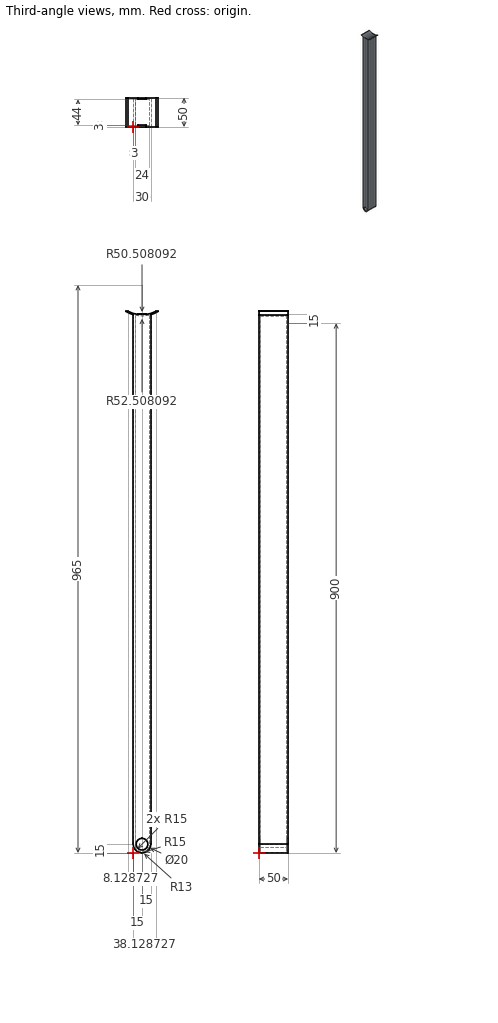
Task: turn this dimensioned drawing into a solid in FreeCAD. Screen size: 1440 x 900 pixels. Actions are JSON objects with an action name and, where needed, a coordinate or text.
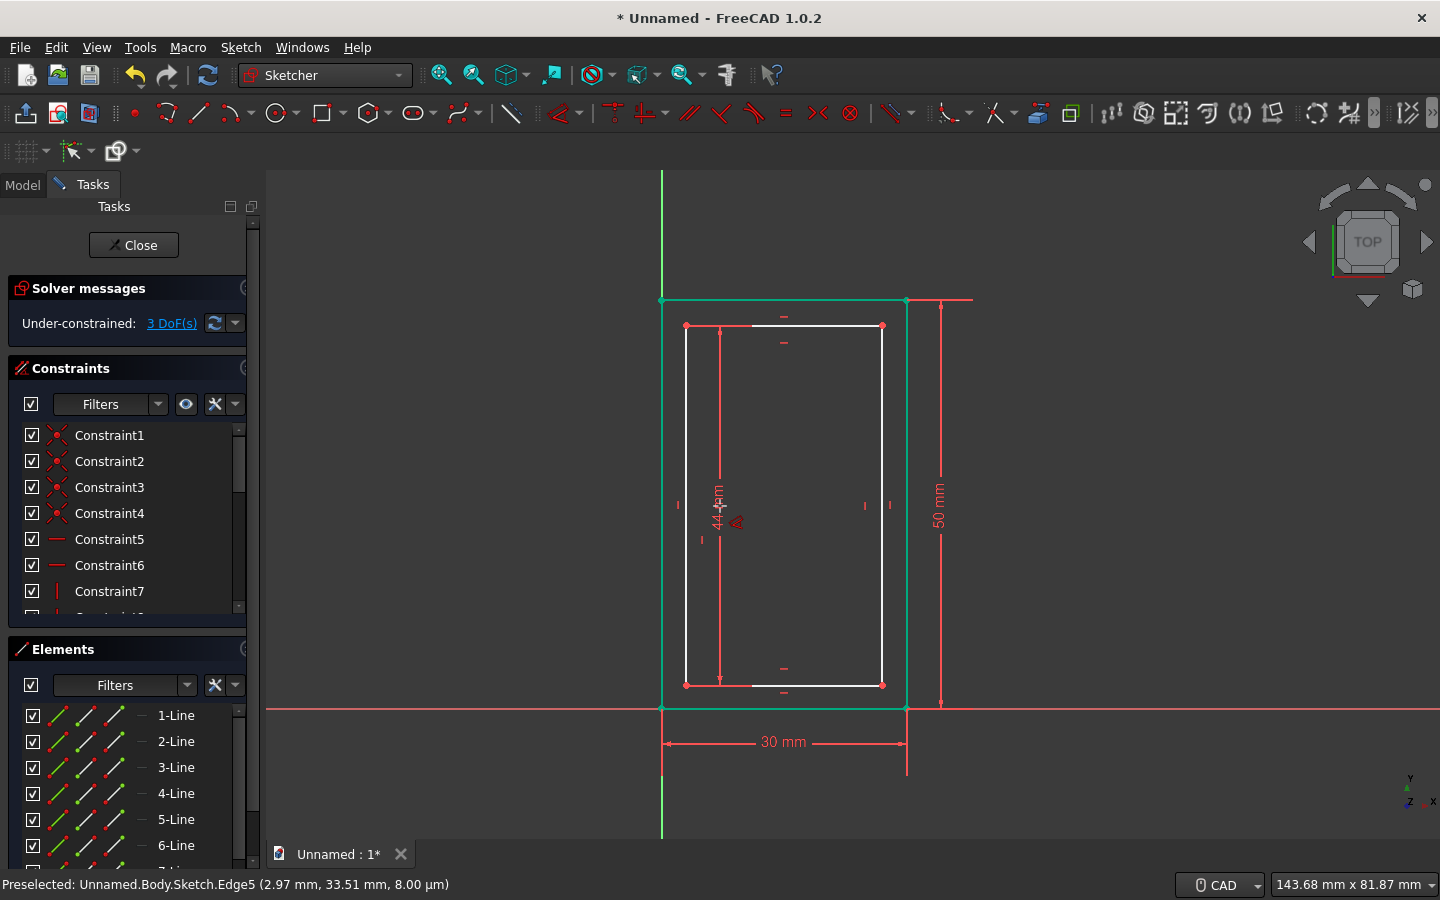
{"action": "left_click", "coordinate": [745, 686]}
{"action": "left_click", "coordinate": [784, 652]}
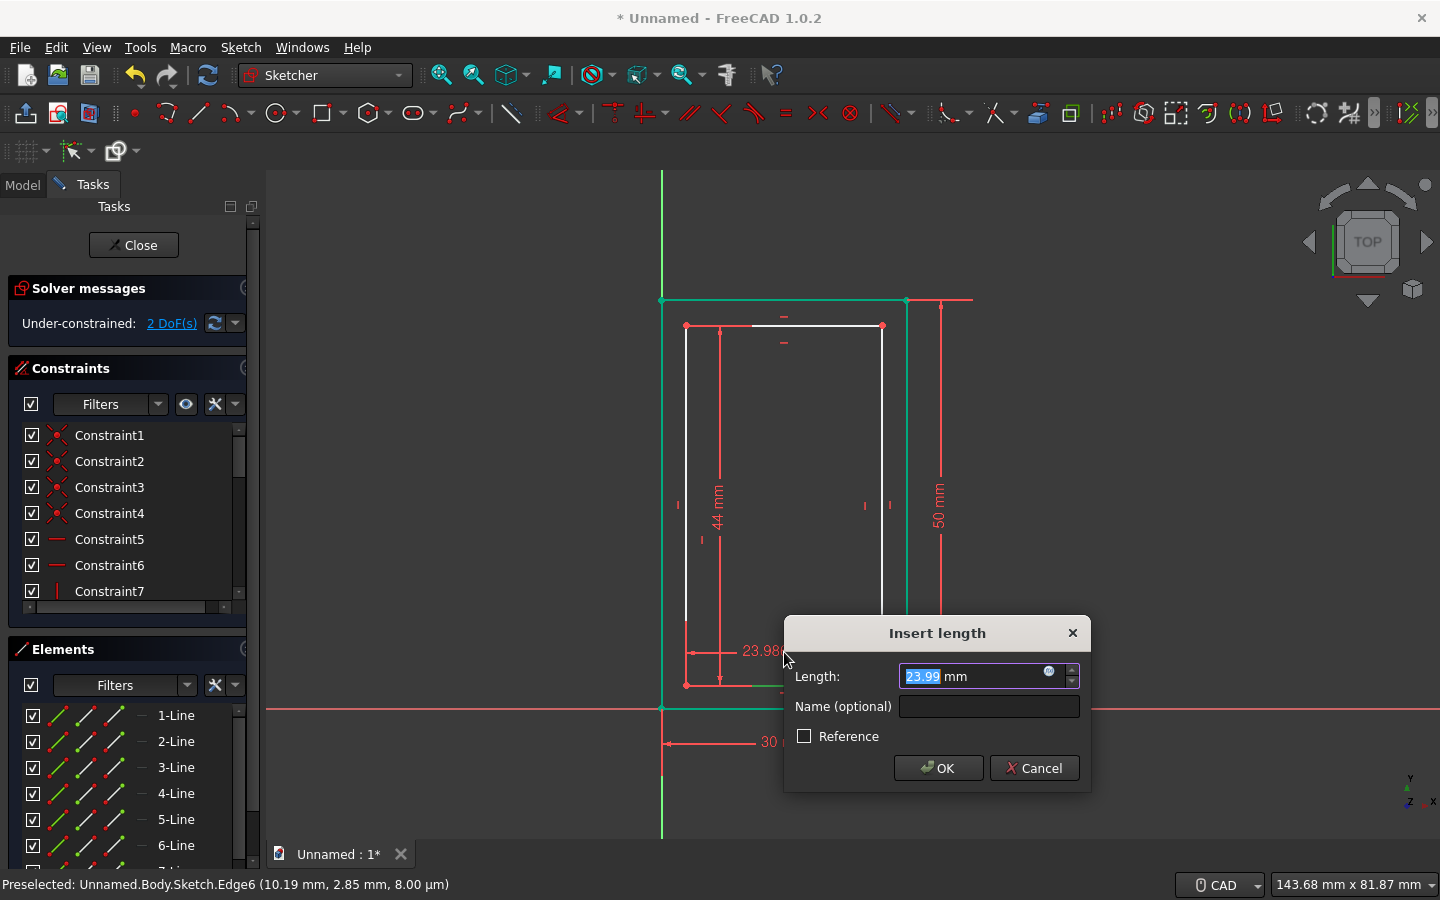
{"action": "type", "text": "24"}
{"action": "key", "text": "Return"}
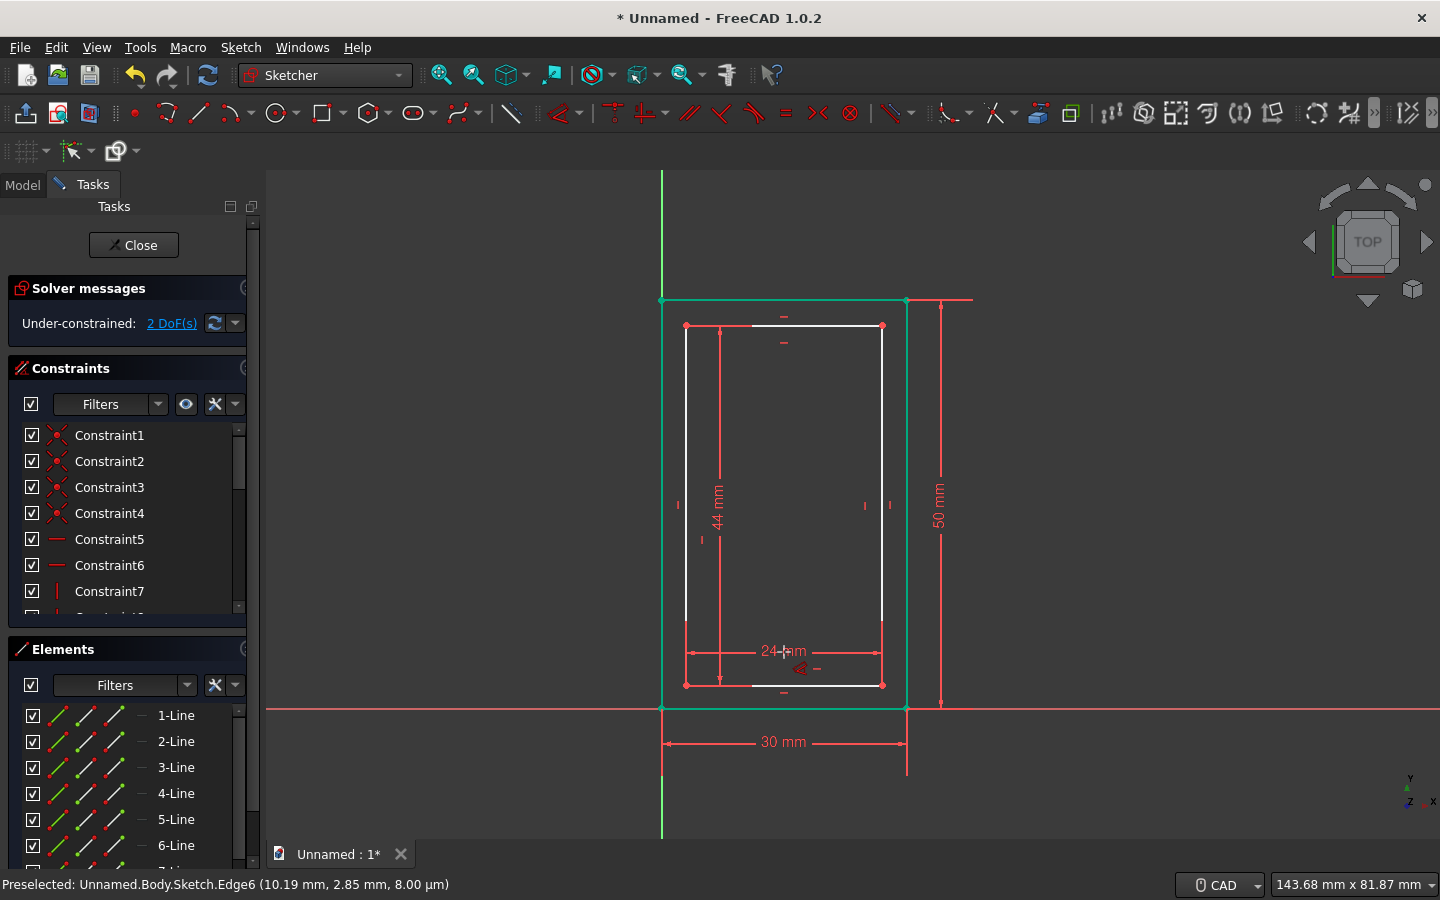
{"action": "scroll", "coordinate": [686, 326], "scroll_direction": "up", "scroll_amount": 3}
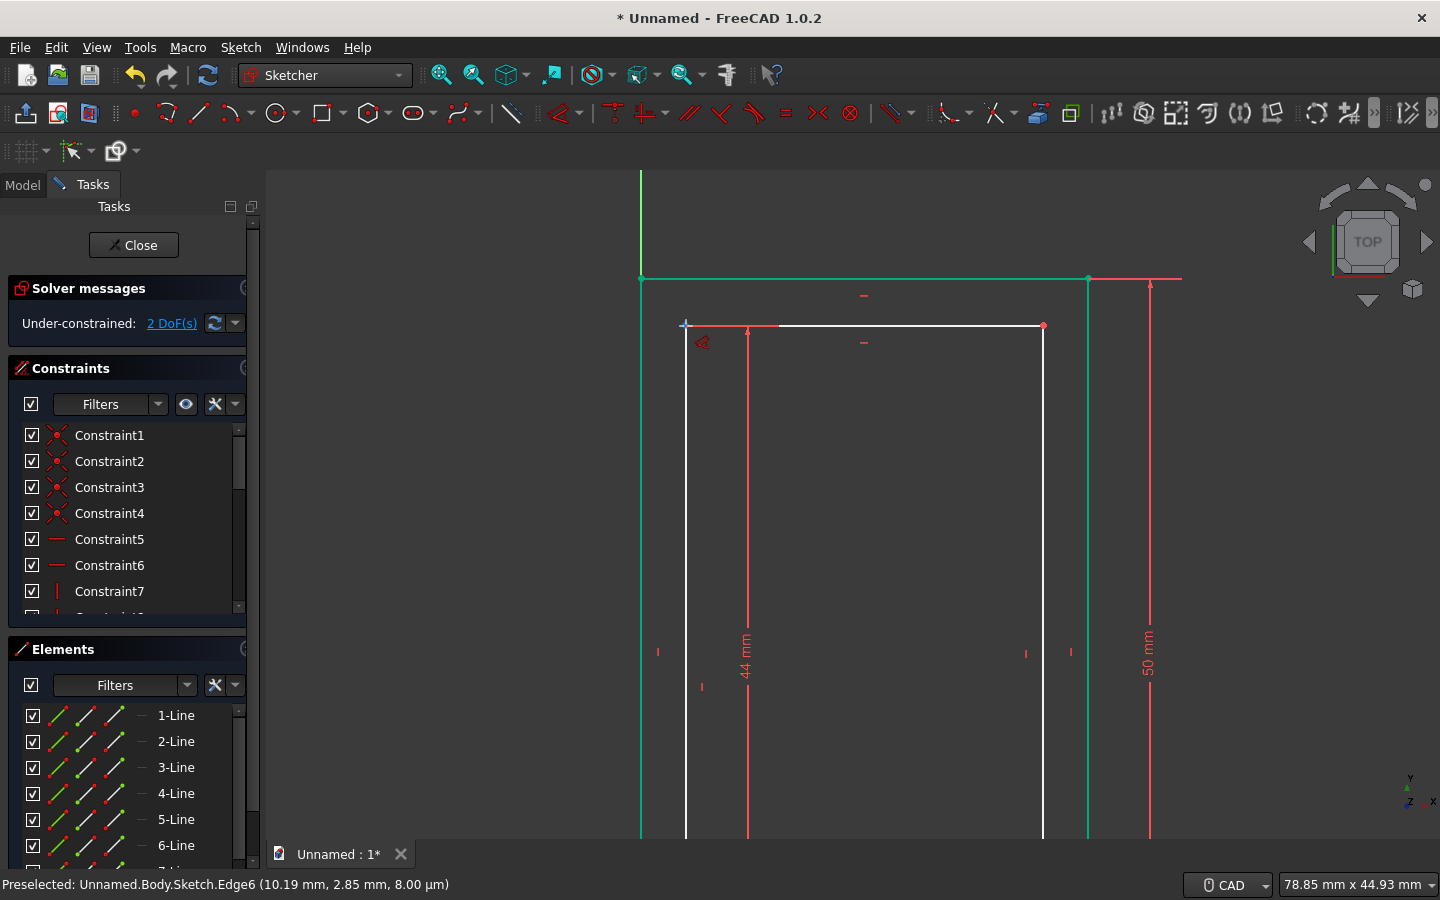
{"action": "left_click", "coordinate": [686, 326]}
{"action": "left_click", "coordinate": [664, 244]}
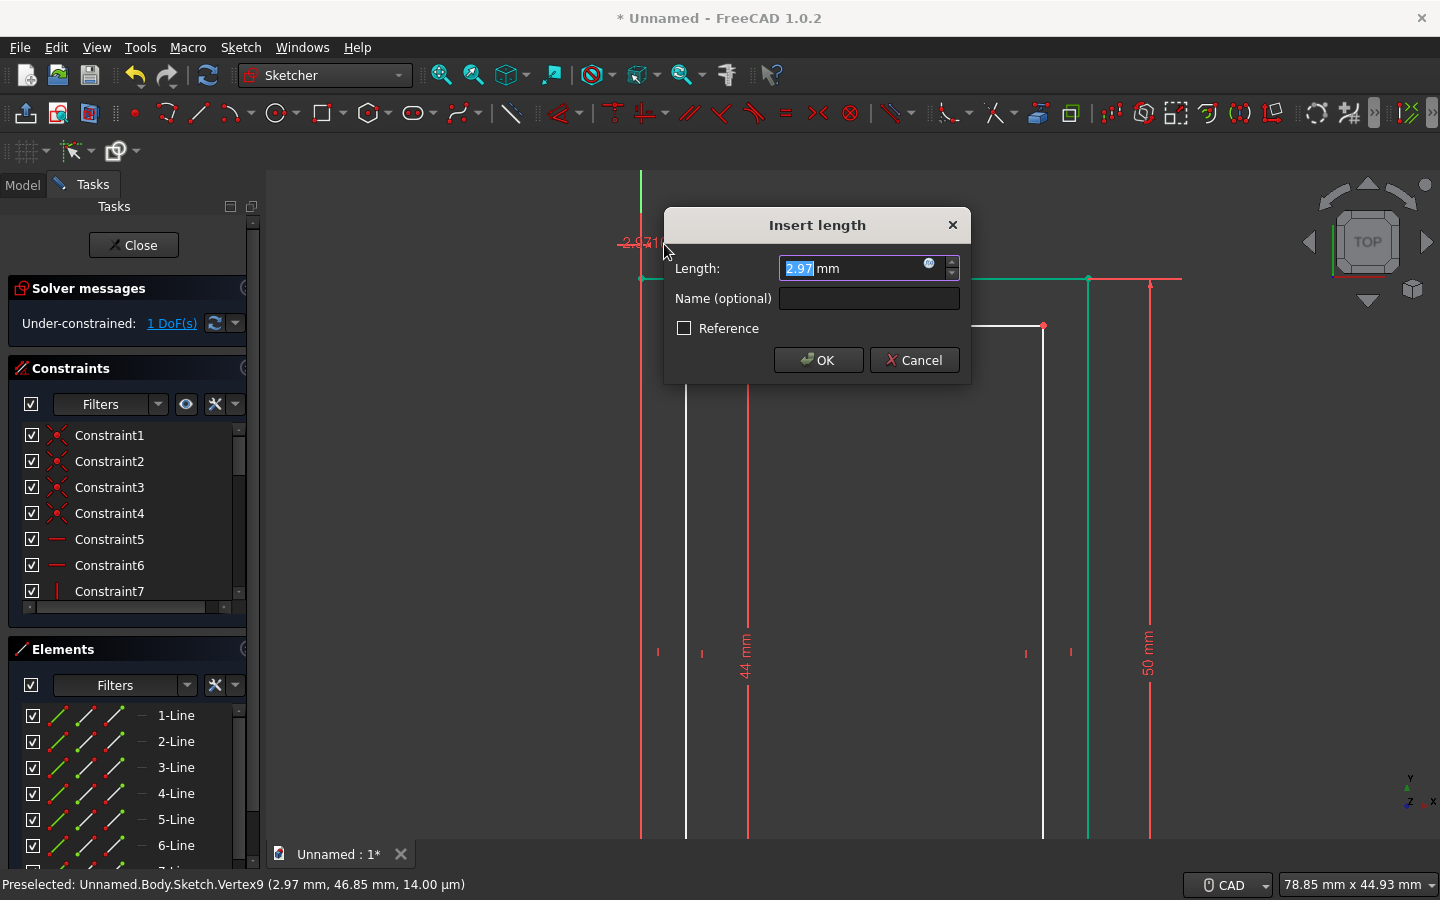
{"action": "type", "text": "3"}
{"action": "key", "text": "Return"}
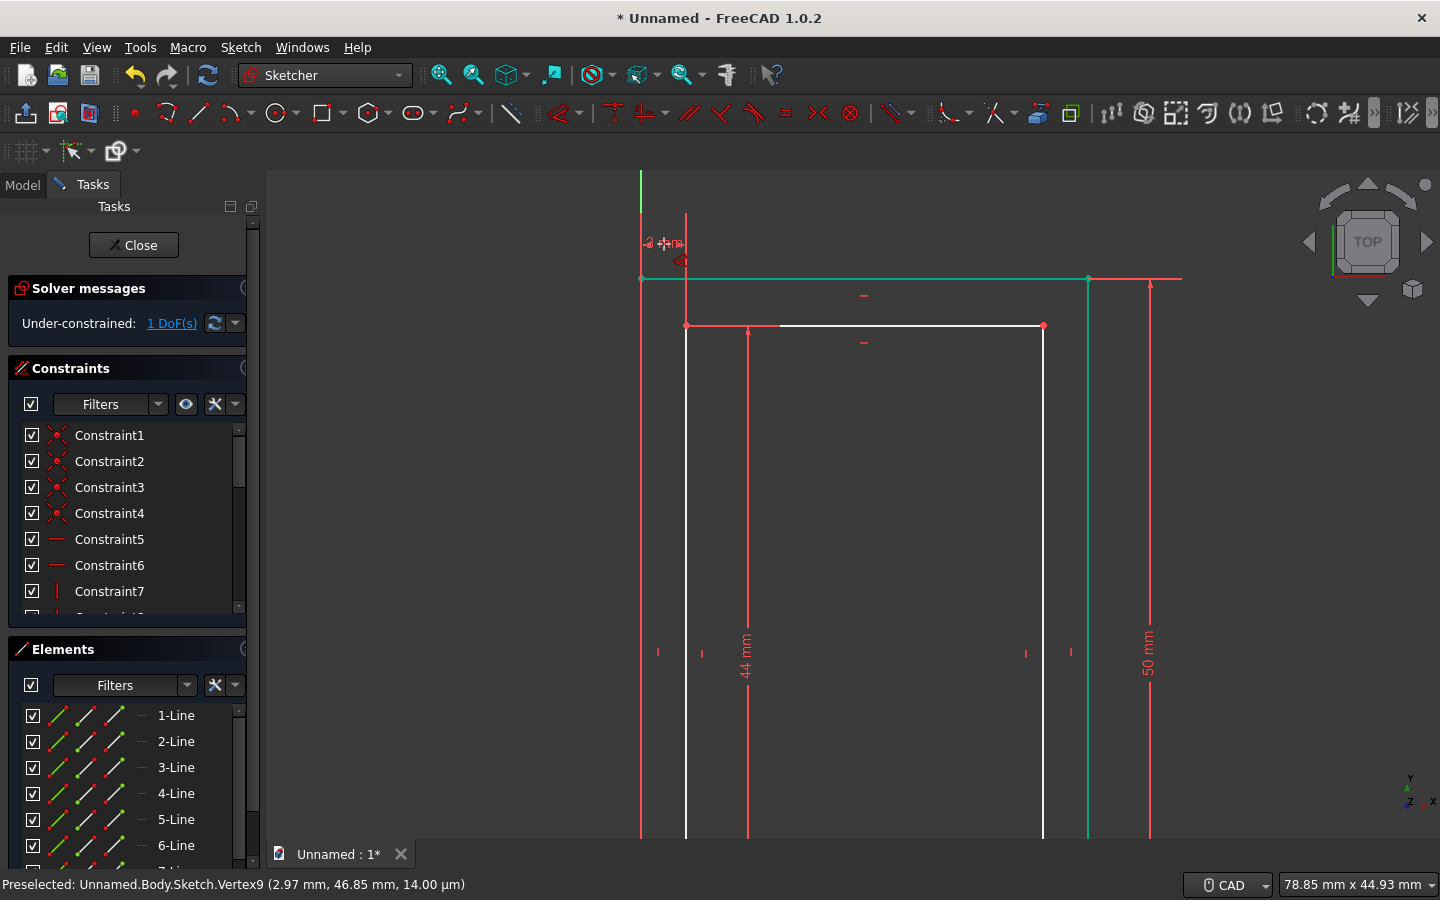
{"action": "scroll", "coordinate": [687, 326], "scroll_direction": "down", "scroll_amount": 3}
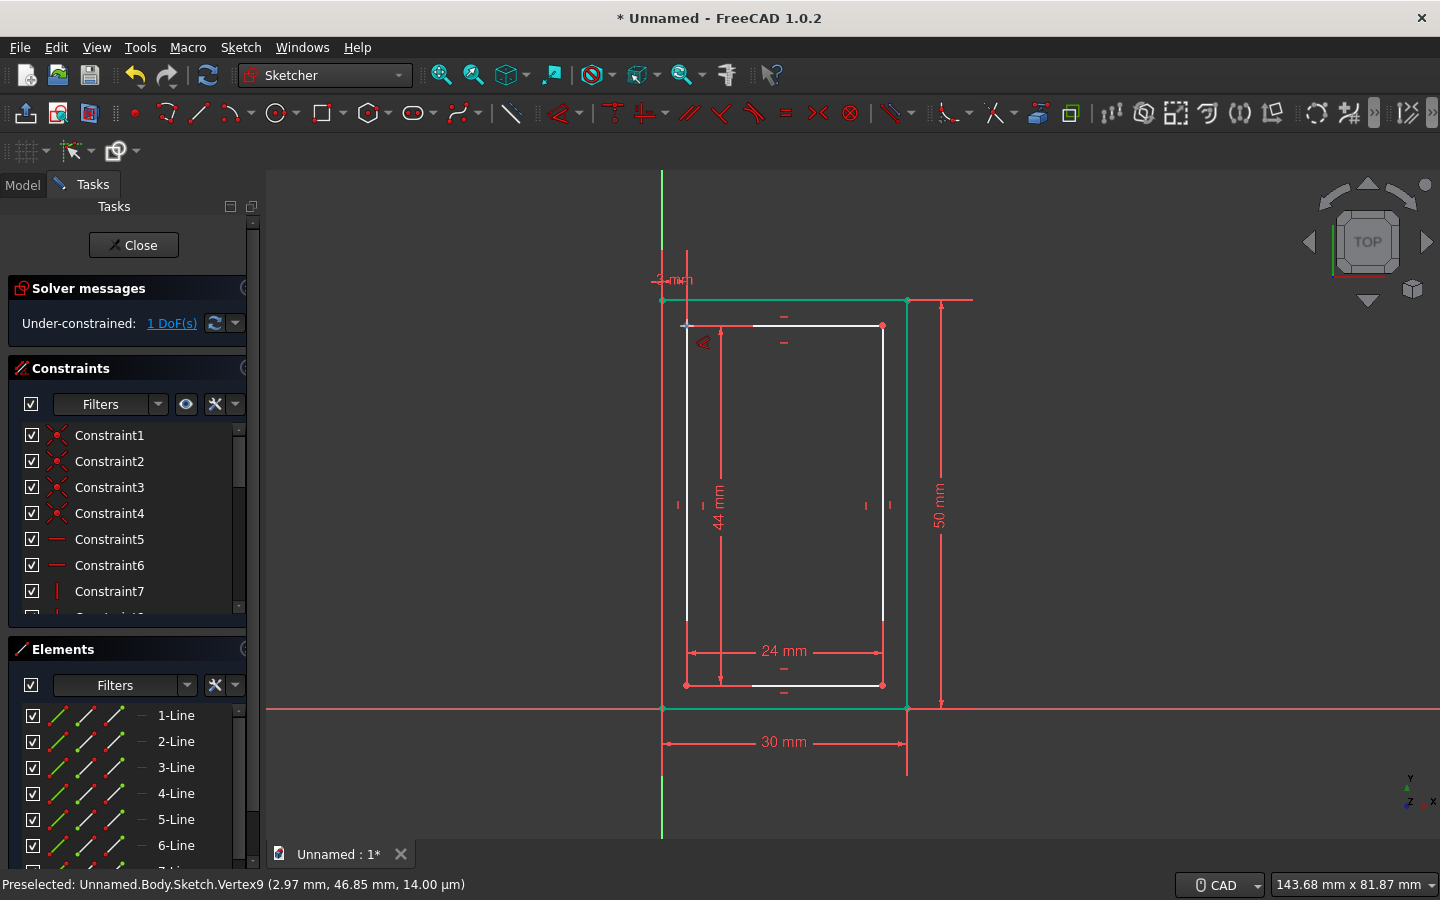
{"action": "scroll", "coordinate": [687, 686], "scroll_direction": "up", "scroll_amount": 3}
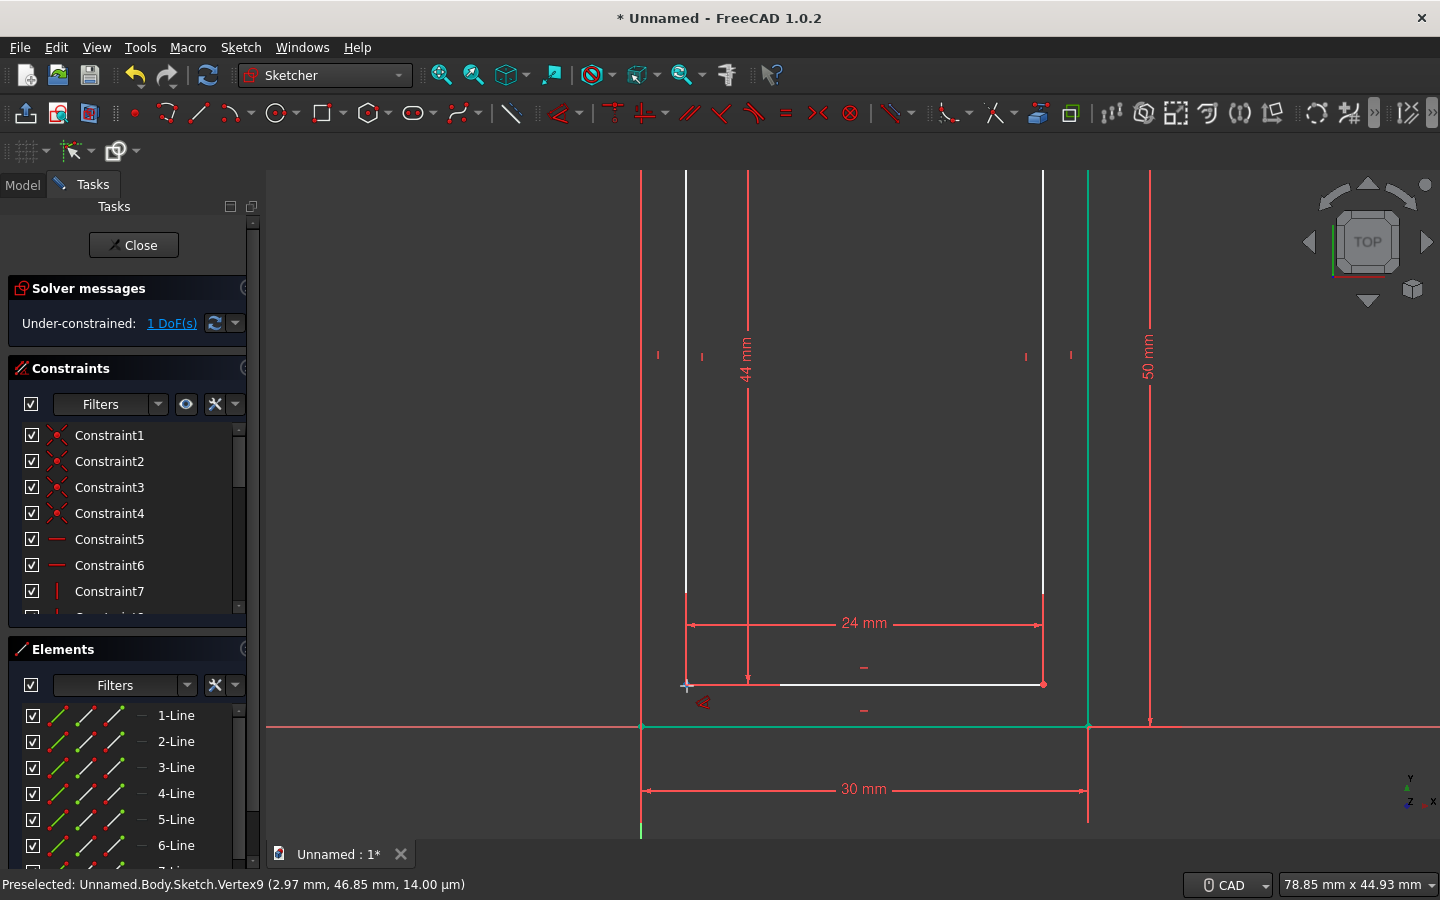
{"action": "left_click", "coordinate": [686, 685]}
{"action": "left_click", "coordinate": [607, 706]}